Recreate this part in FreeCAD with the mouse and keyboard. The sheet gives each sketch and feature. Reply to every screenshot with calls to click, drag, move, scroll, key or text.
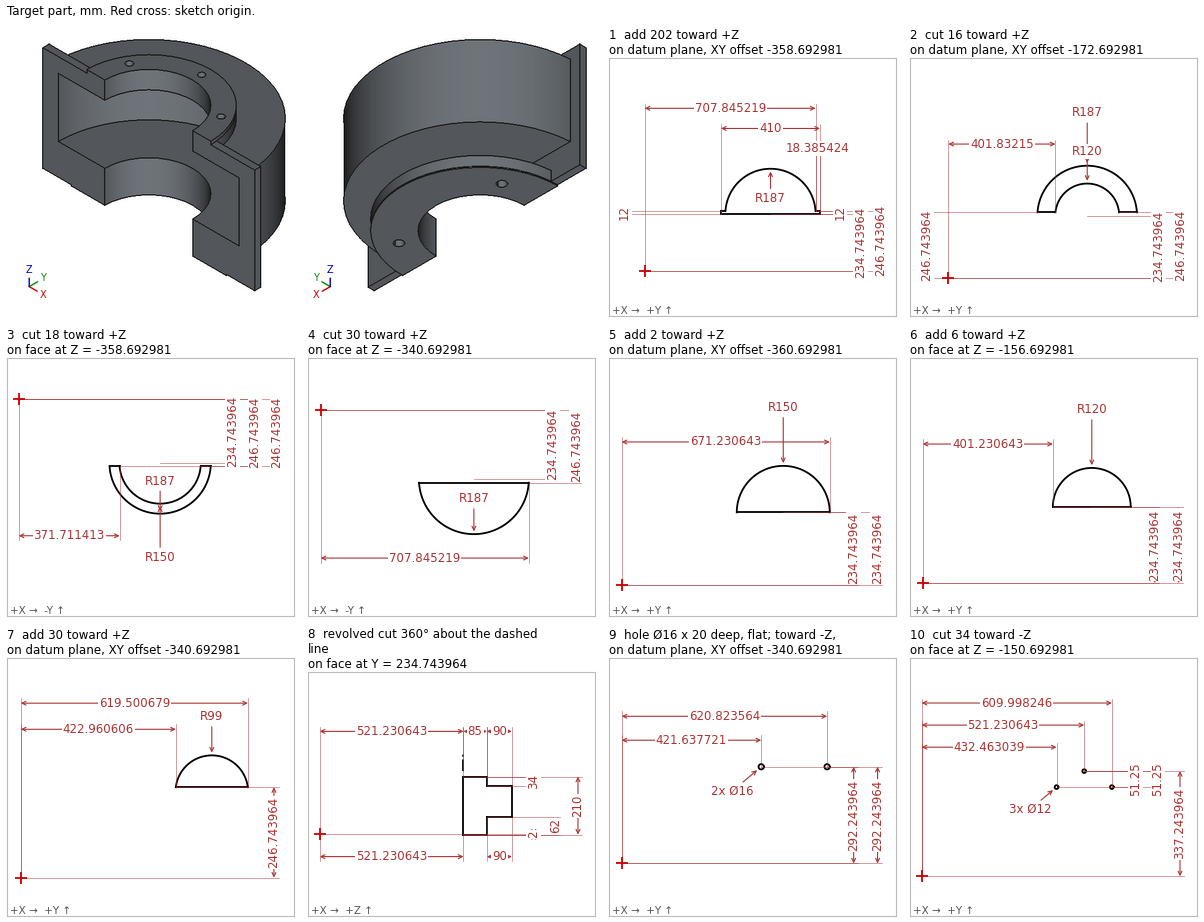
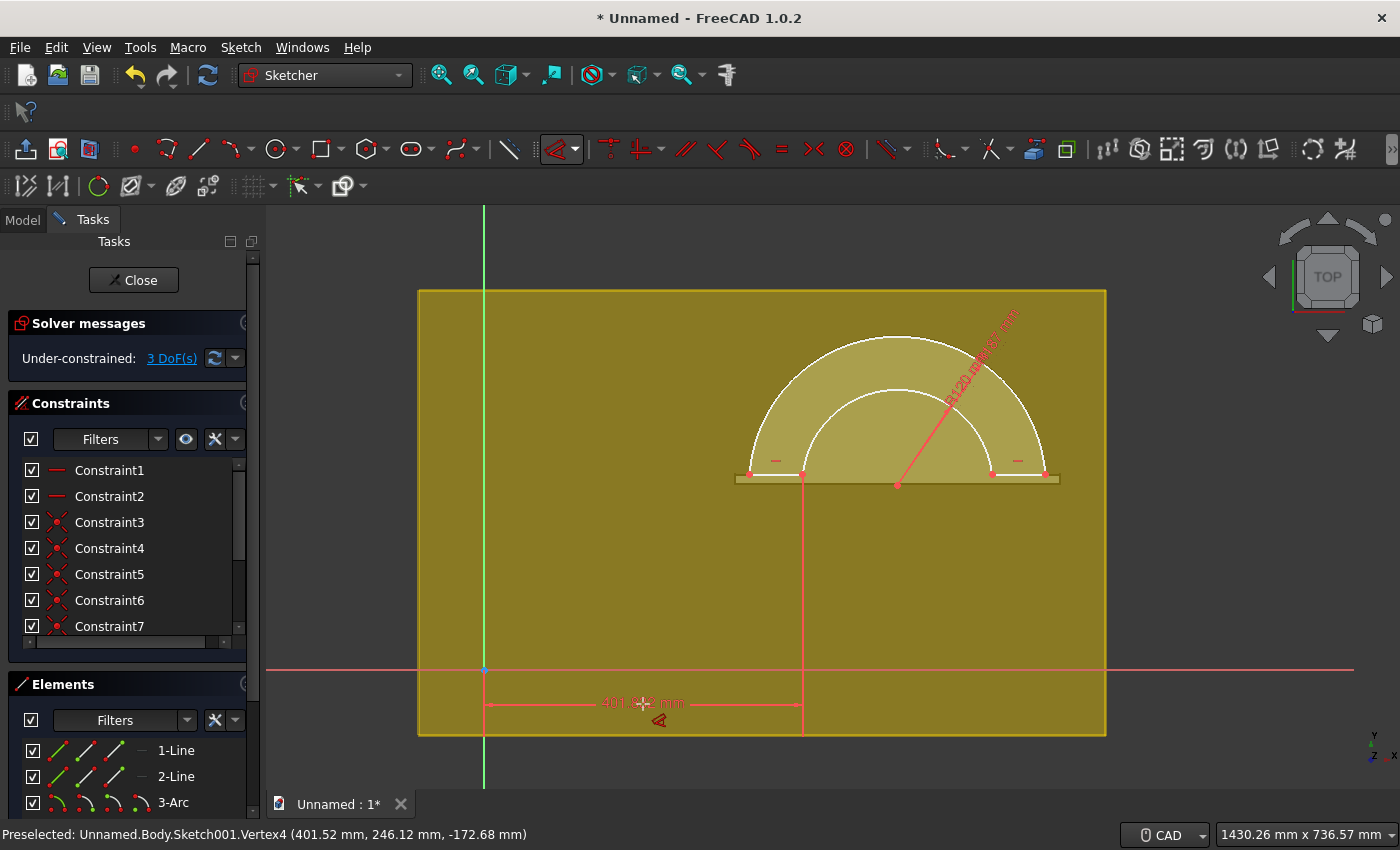
click(992, 475)
click(450, 573)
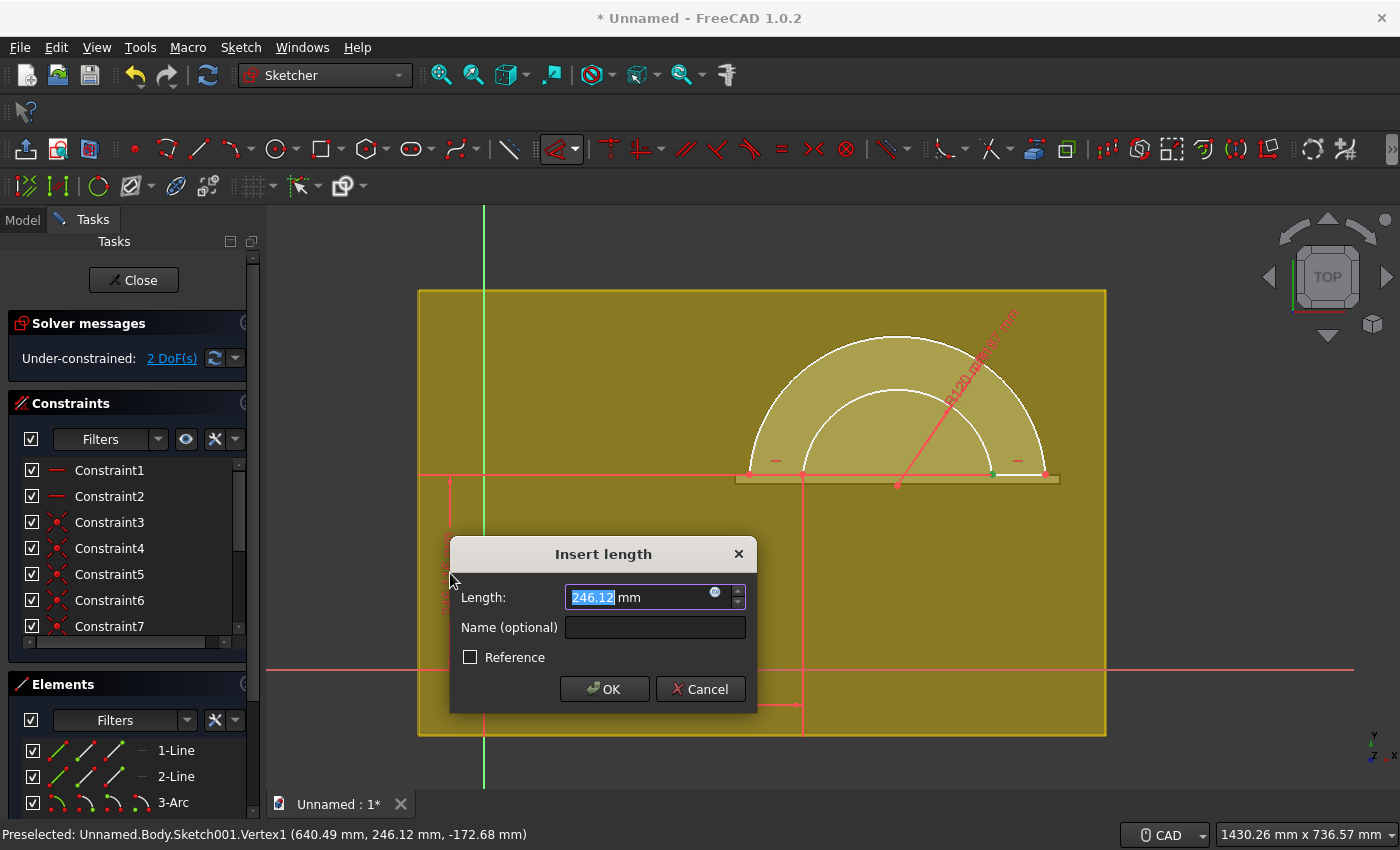
text(246.743964)
key(Return)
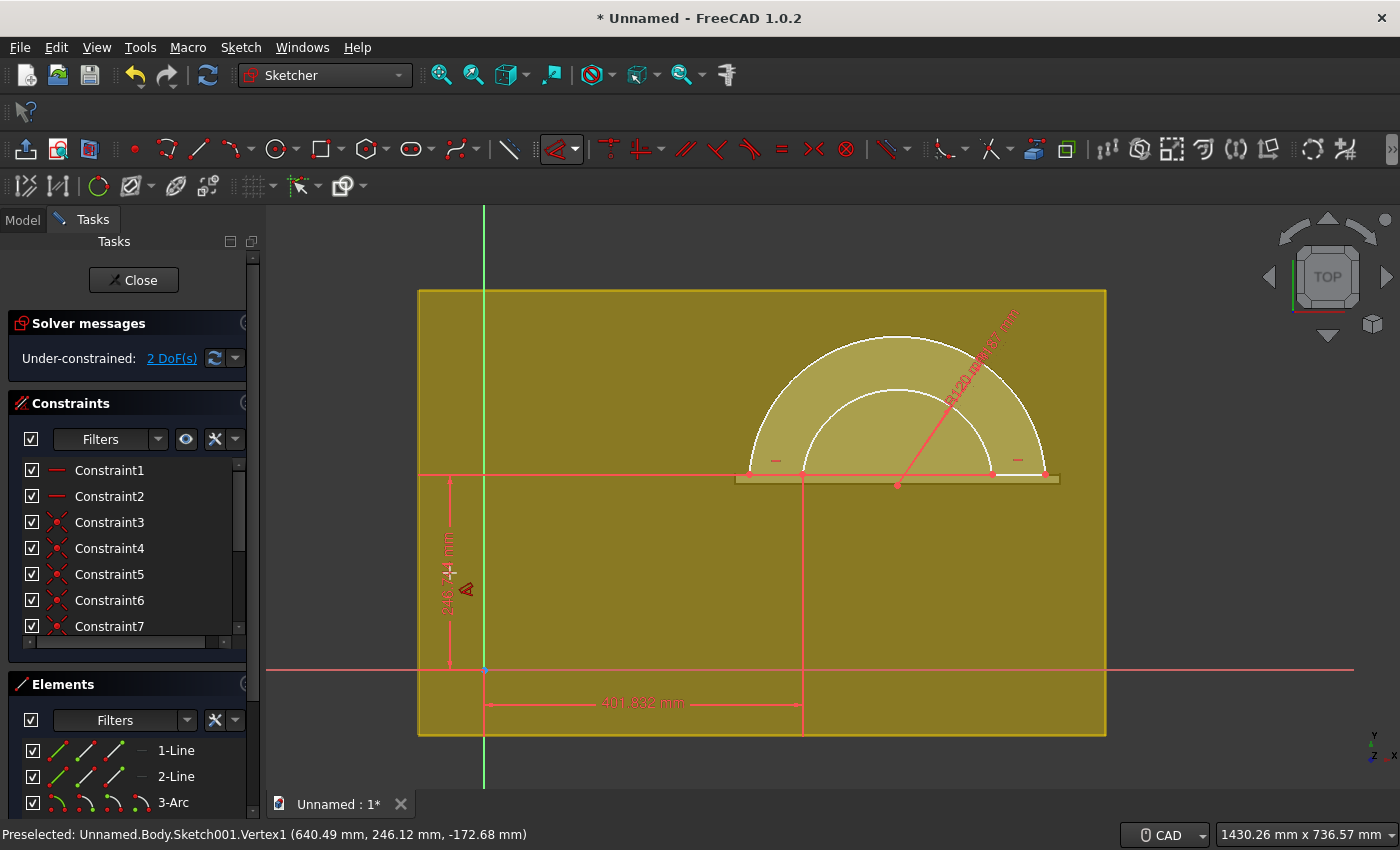
click(750, 475)
click(450, 528)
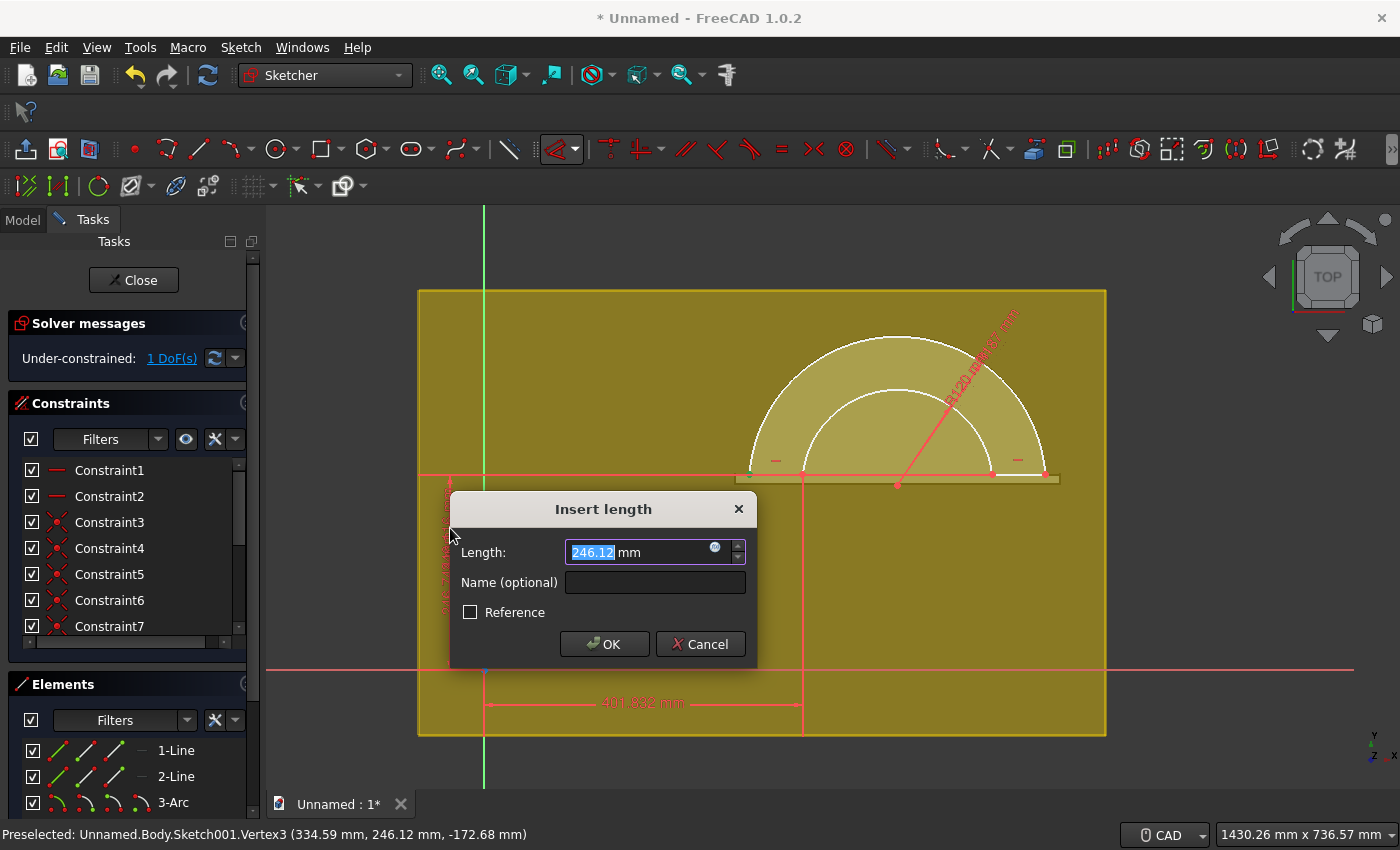
text(246.743964)
key(Return)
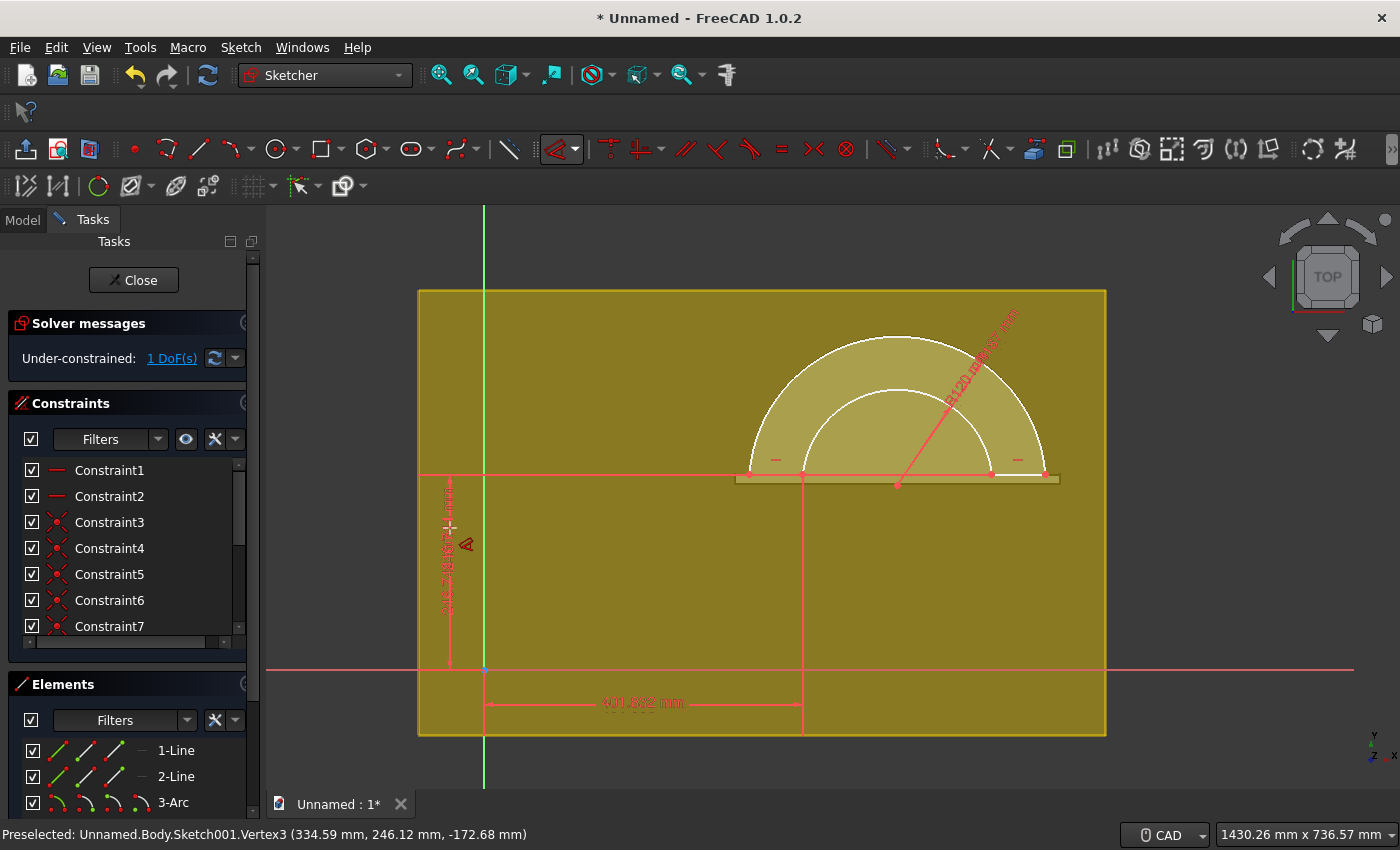
click(897, 485)
click(450, 620)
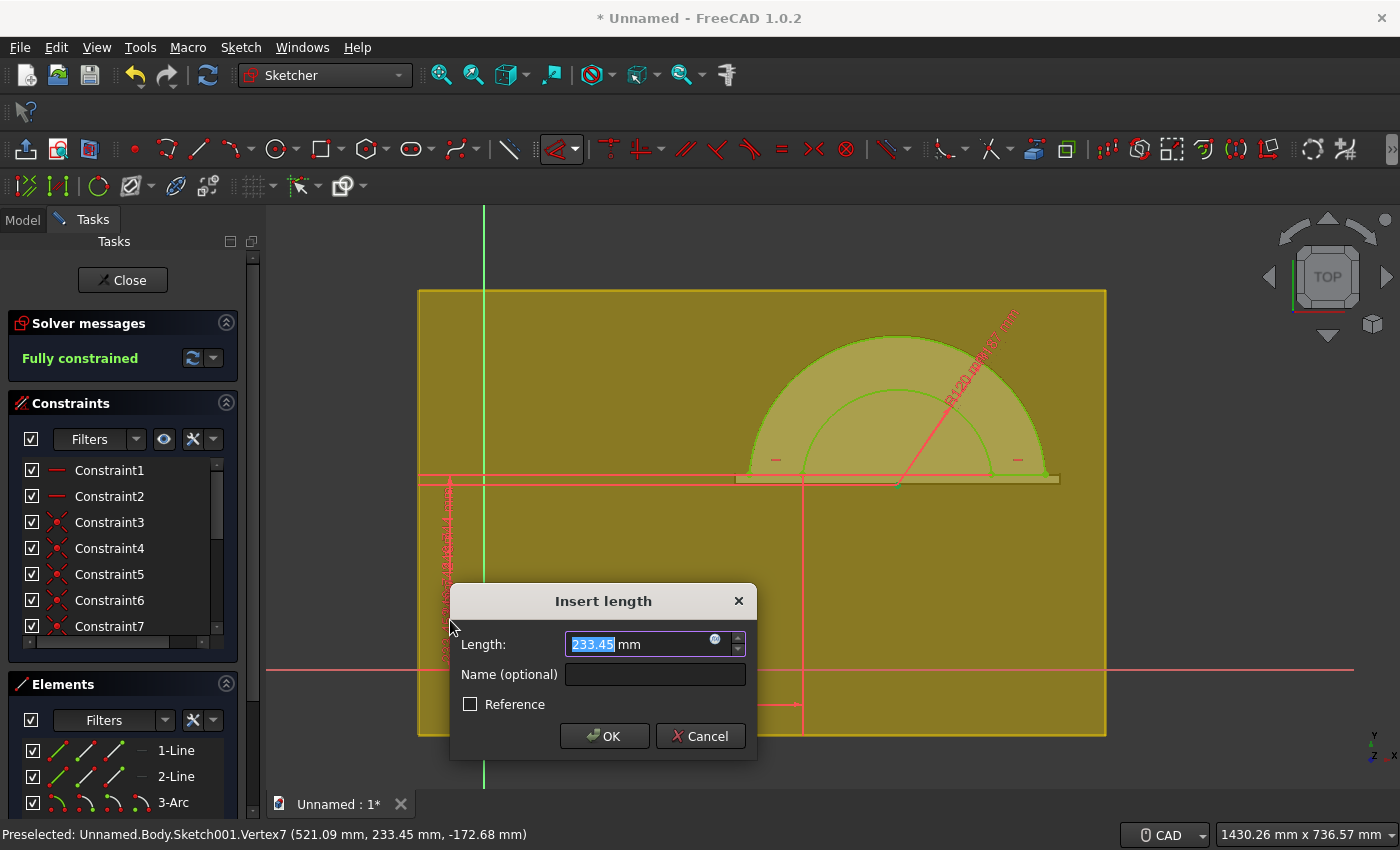
text(234.743964)
key(Return)
key(Escape)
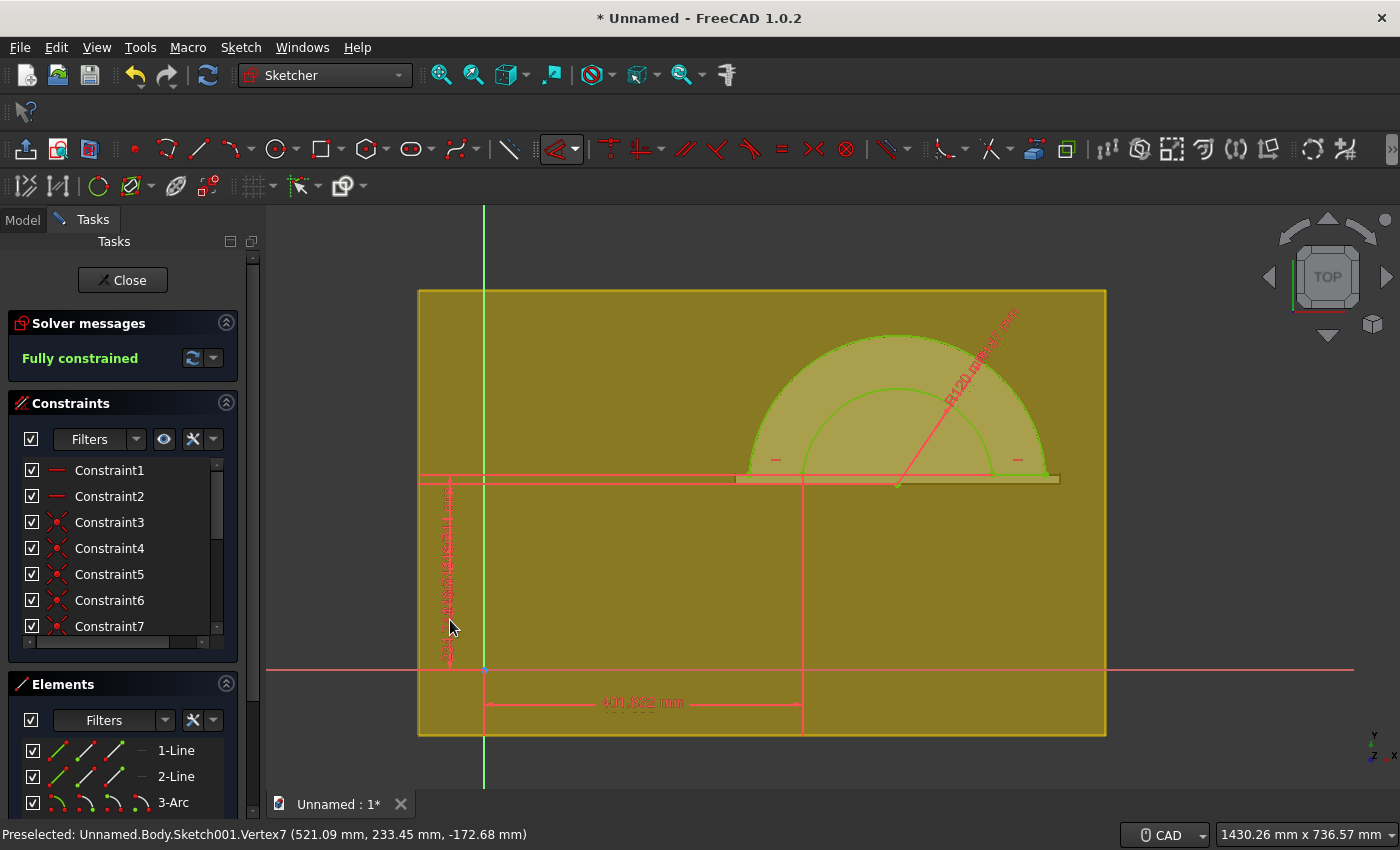
click(123, 280)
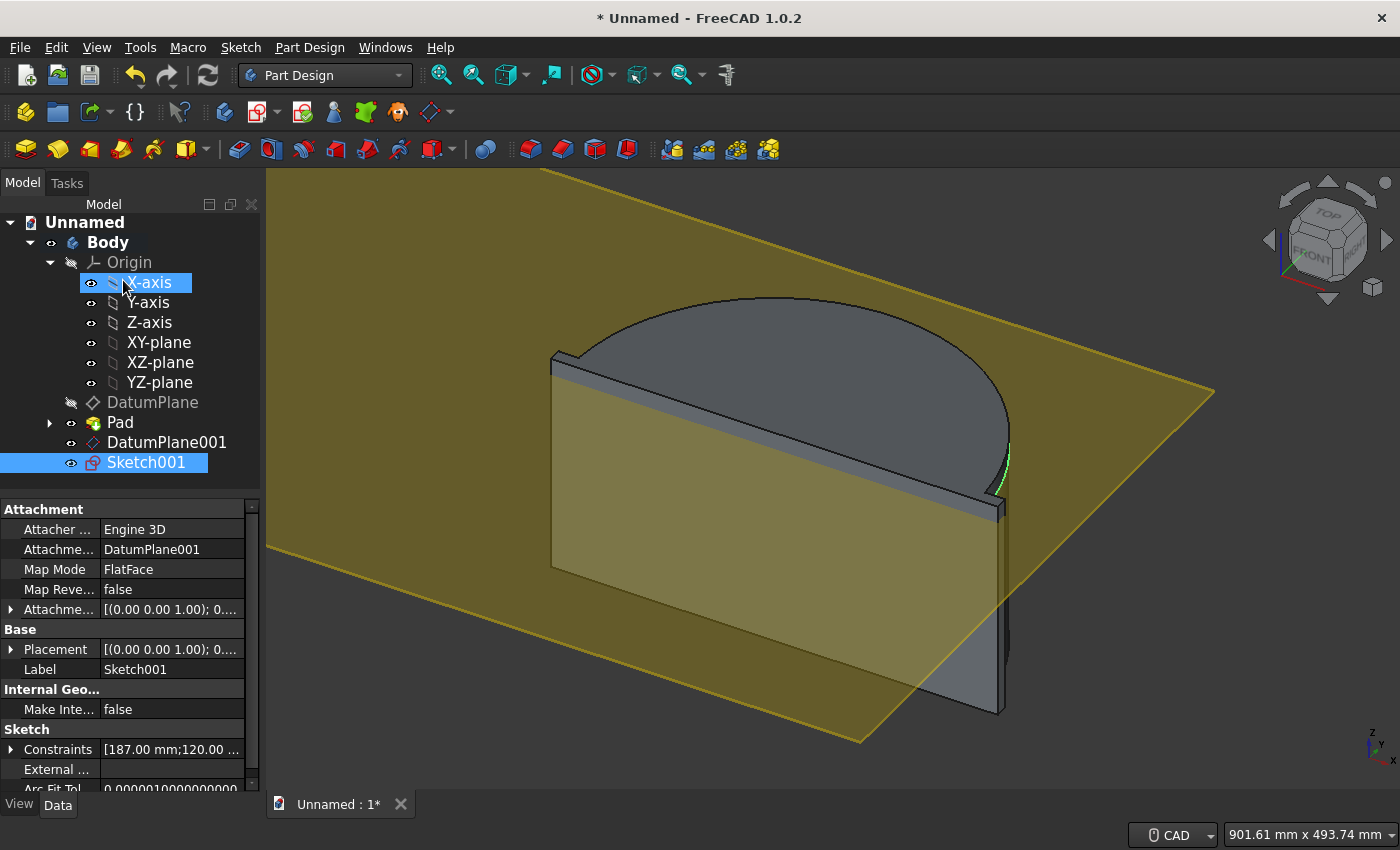
click(240, 150)